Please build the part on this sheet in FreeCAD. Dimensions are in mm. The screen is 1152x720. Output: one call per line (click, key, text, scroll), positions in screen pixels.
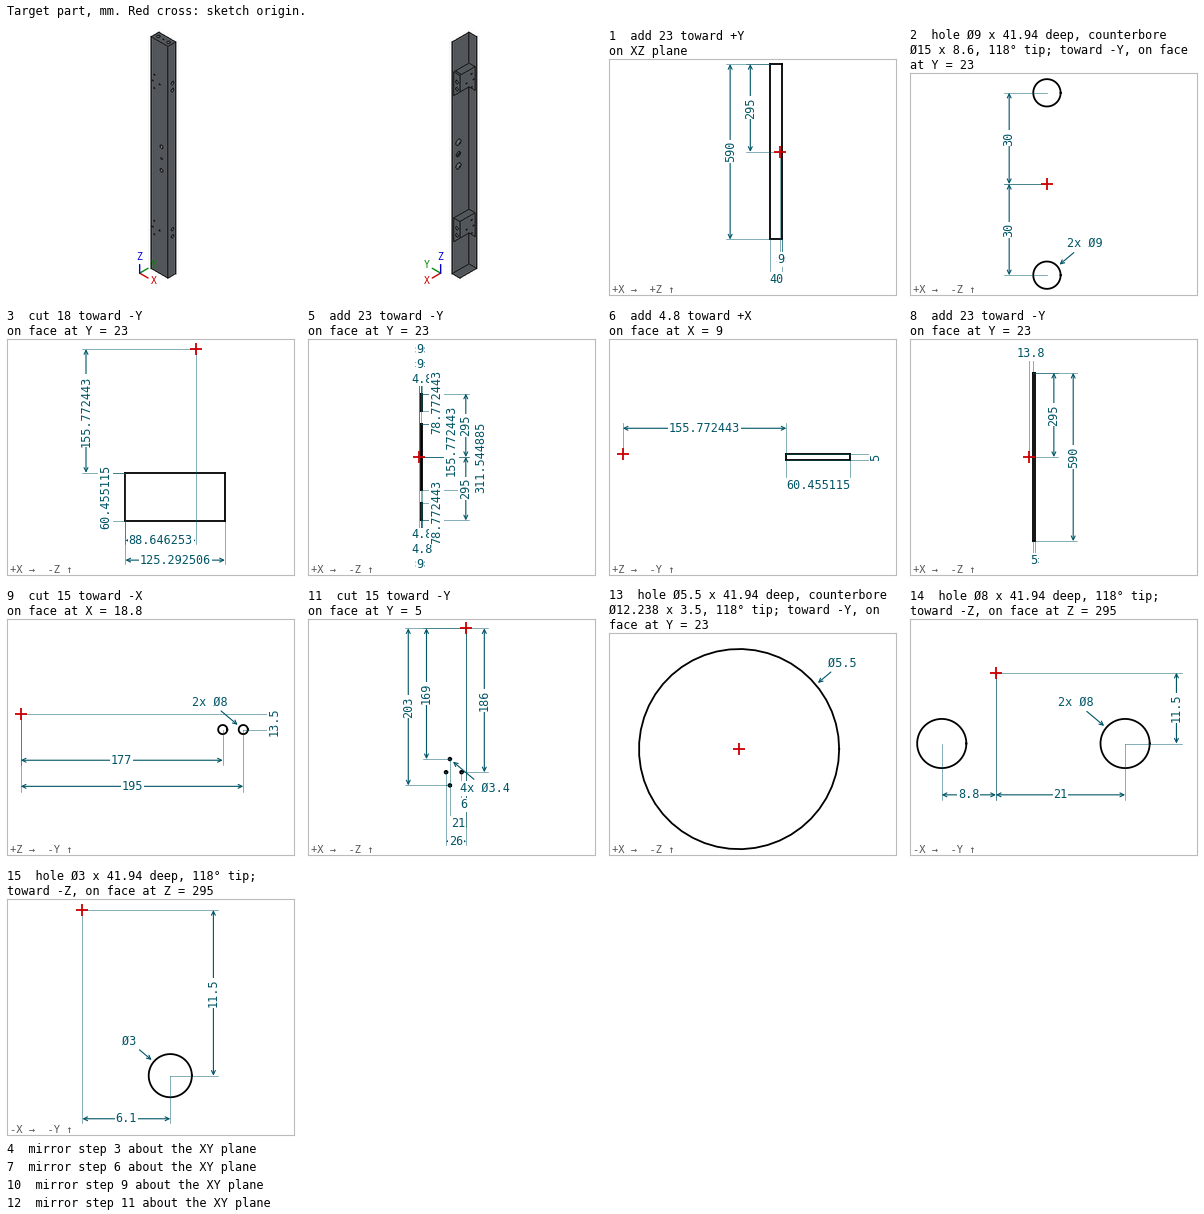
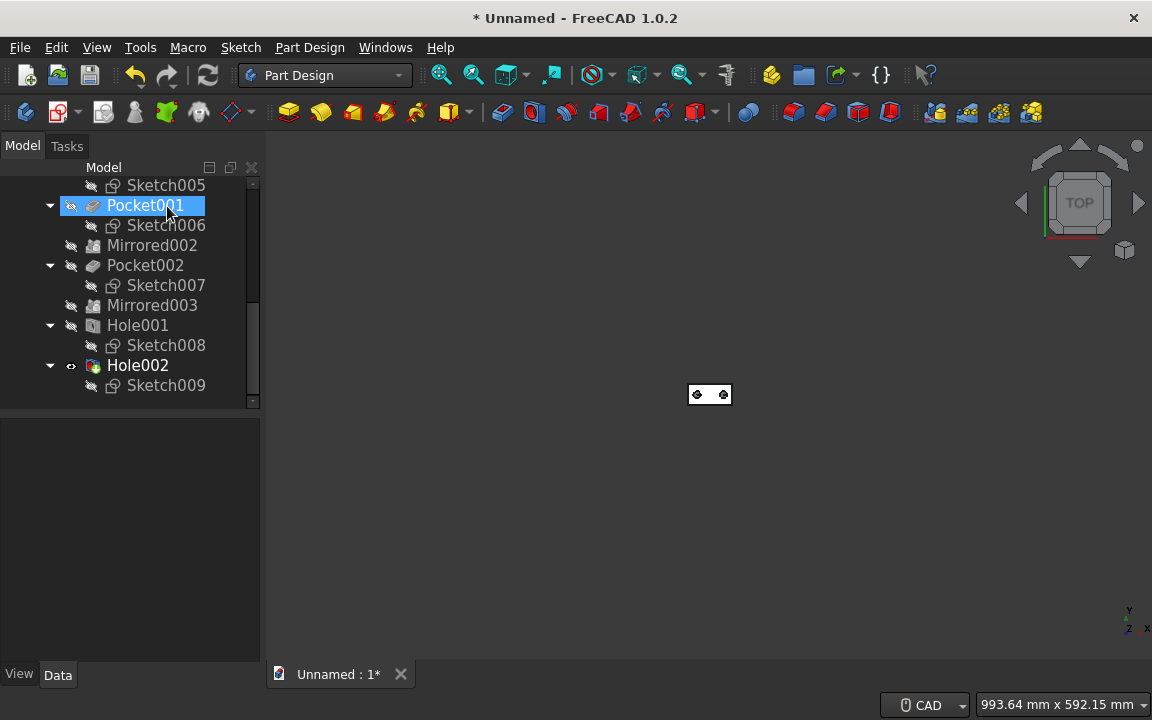
click(442, 76)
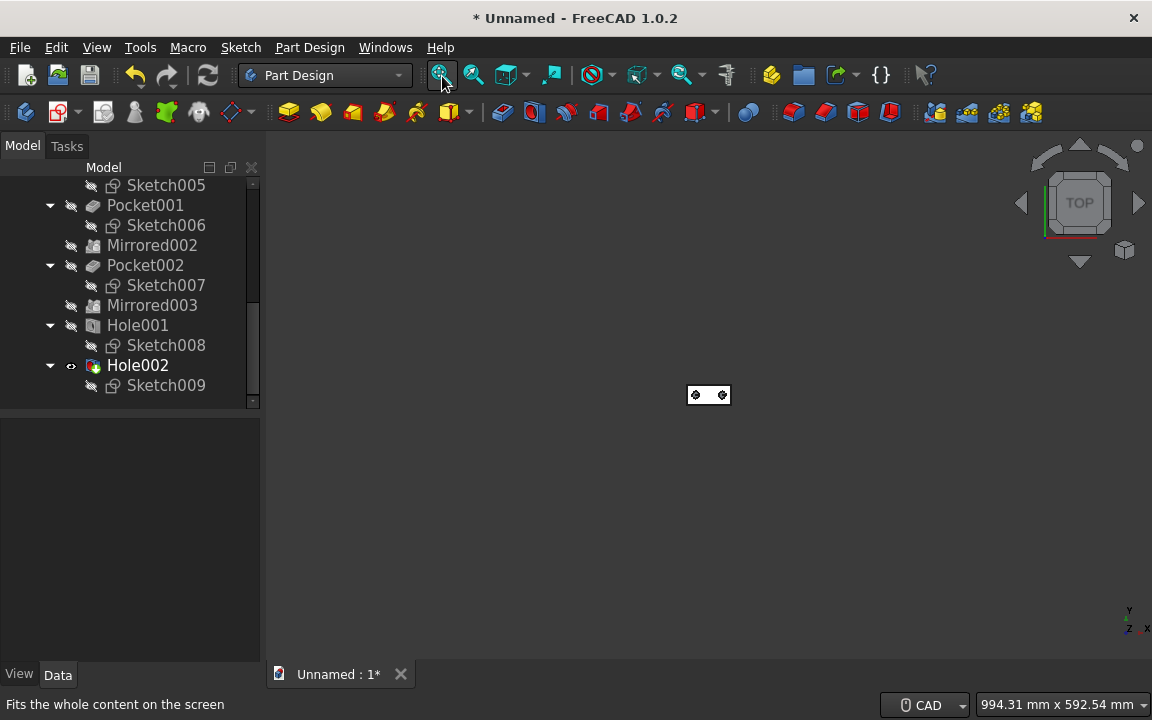
click(709, 394)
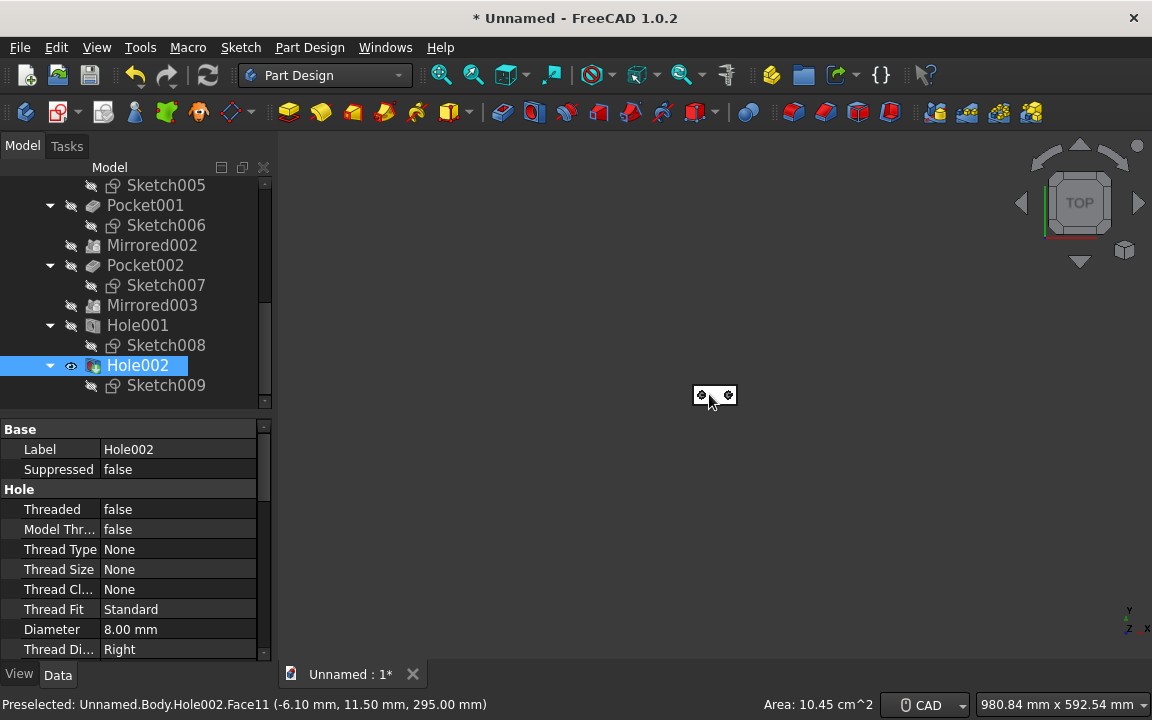
click(58, 112)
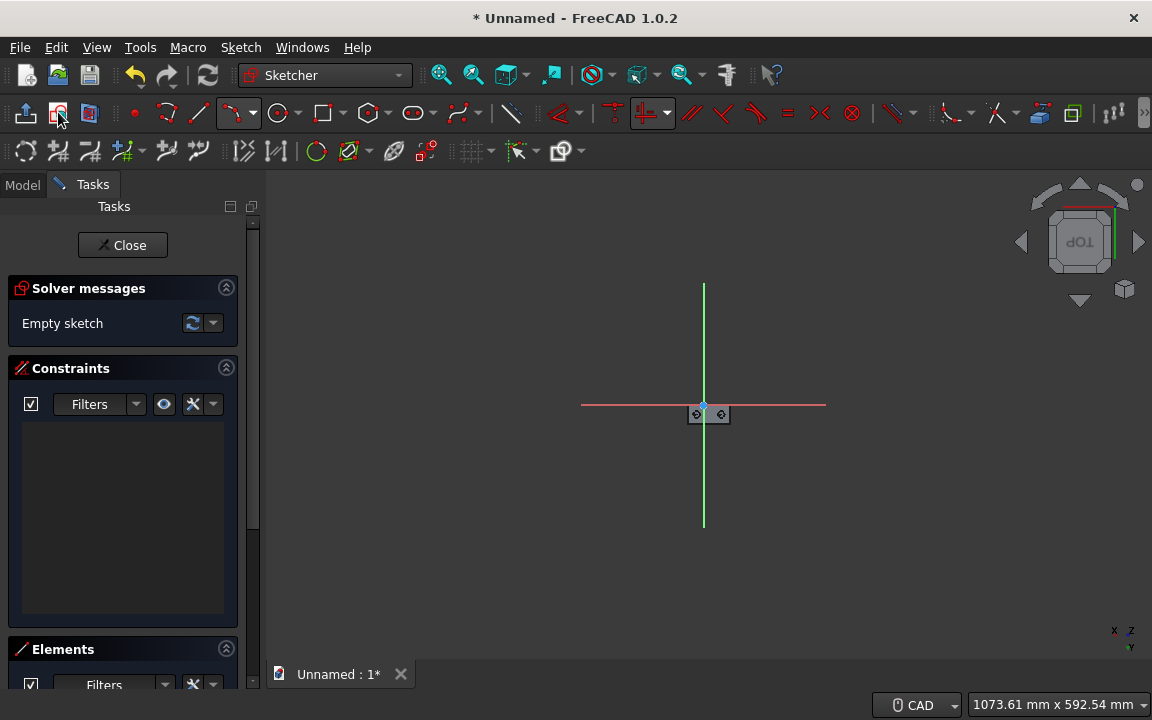
scroll(713, 414, up, 15)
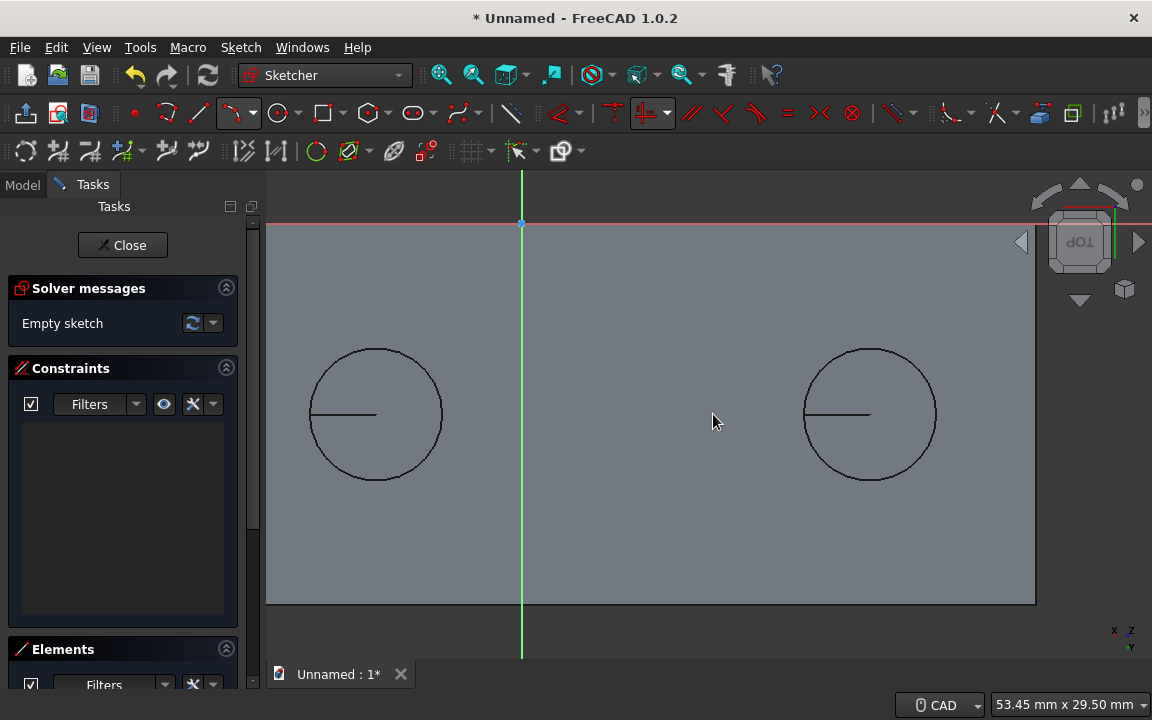
scroll(620, 414, up, 9)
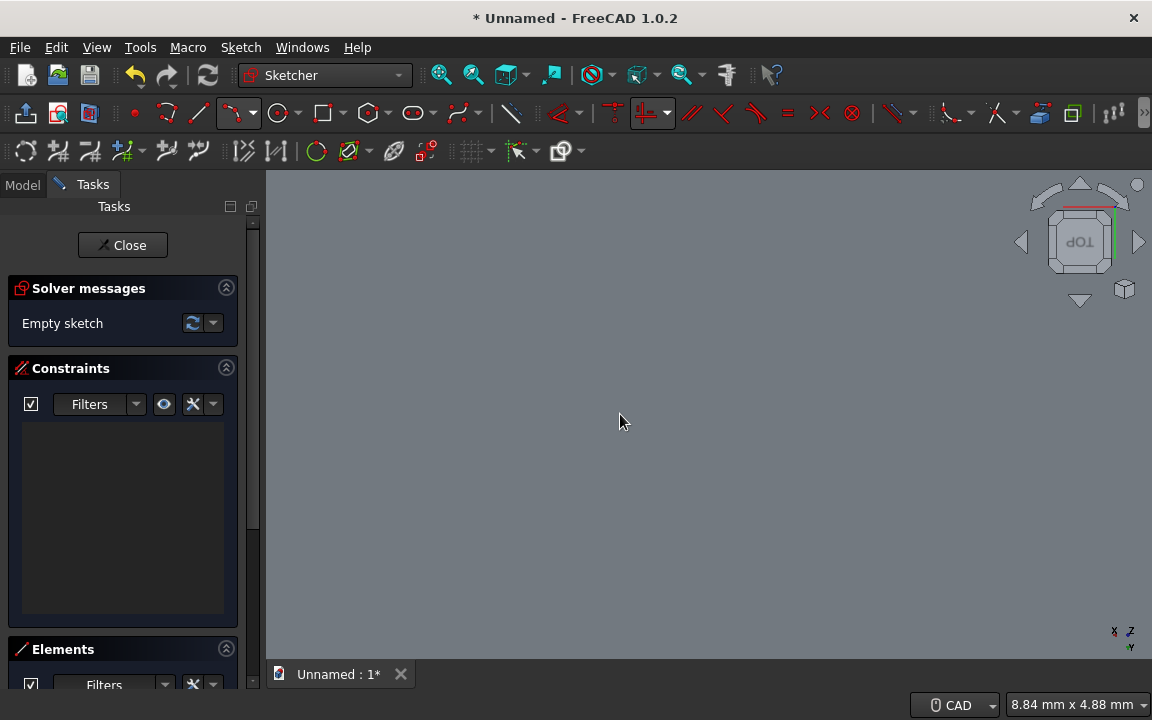
click(278, 114)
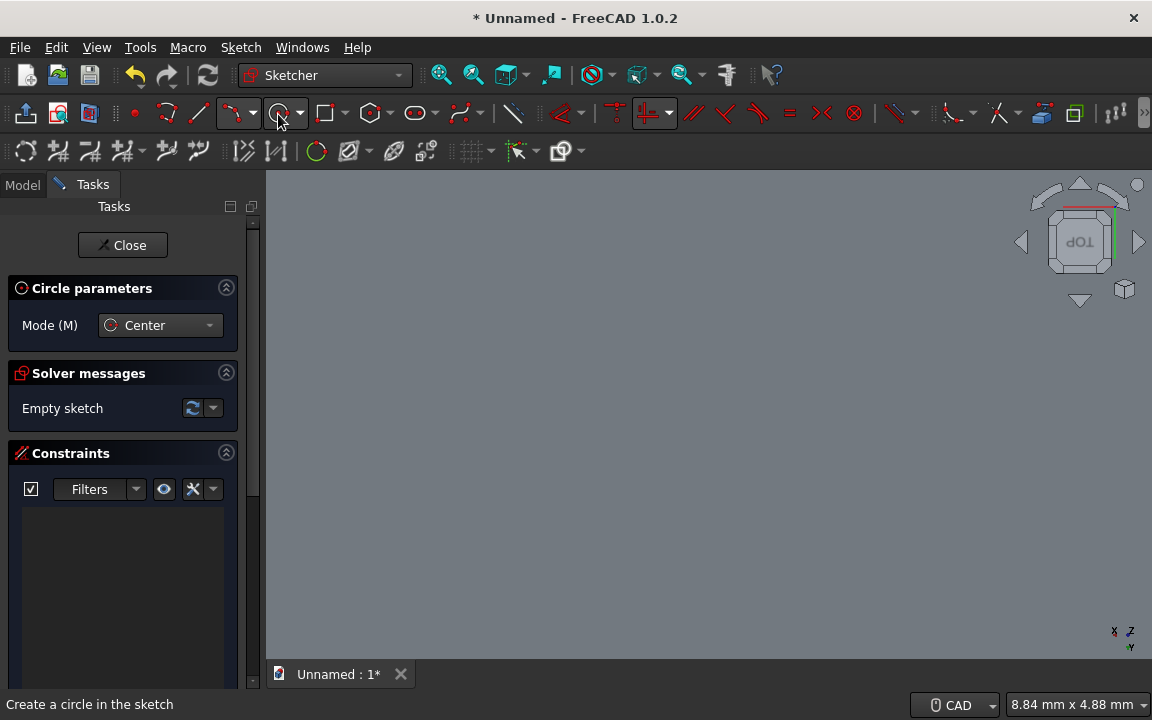
click(636, 414)
click(743, 308)
key(Escape)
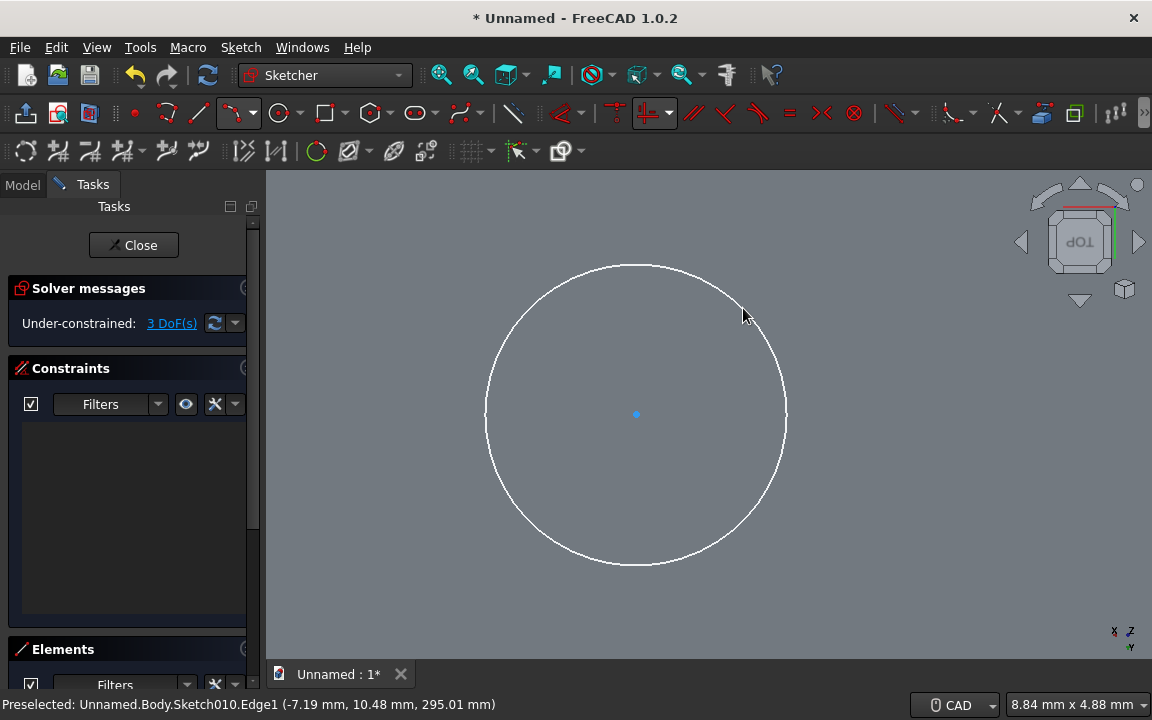
click(560, 114)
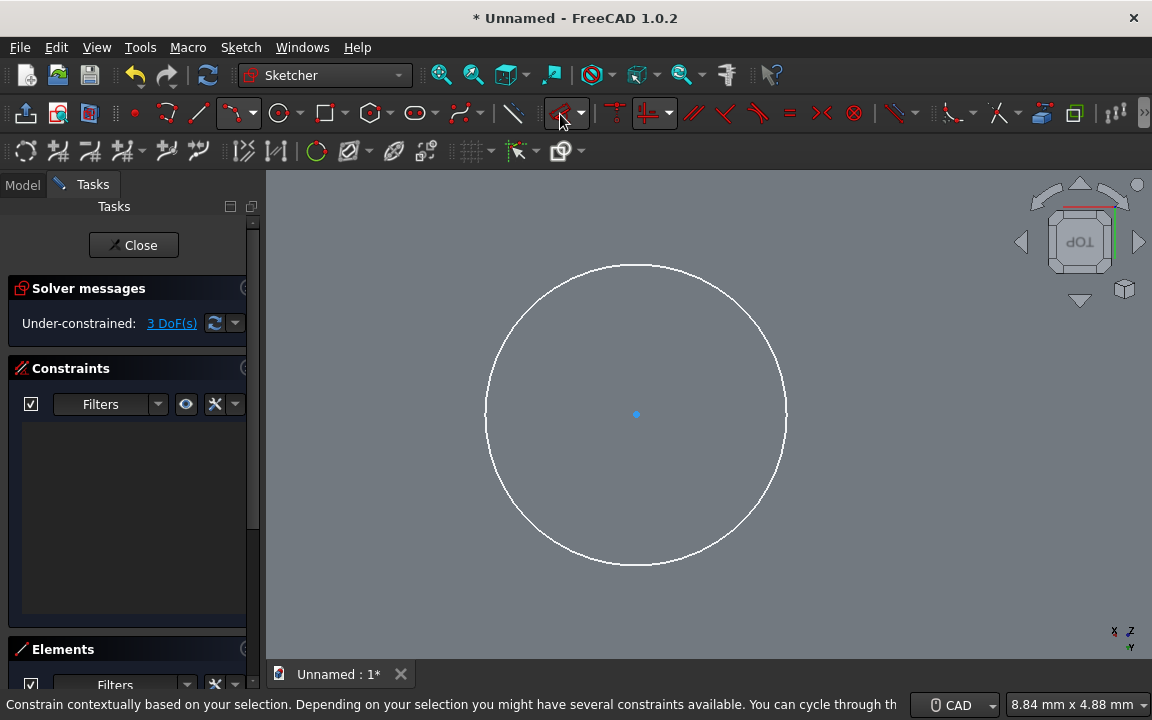
click(742, 308)
click(765, 285)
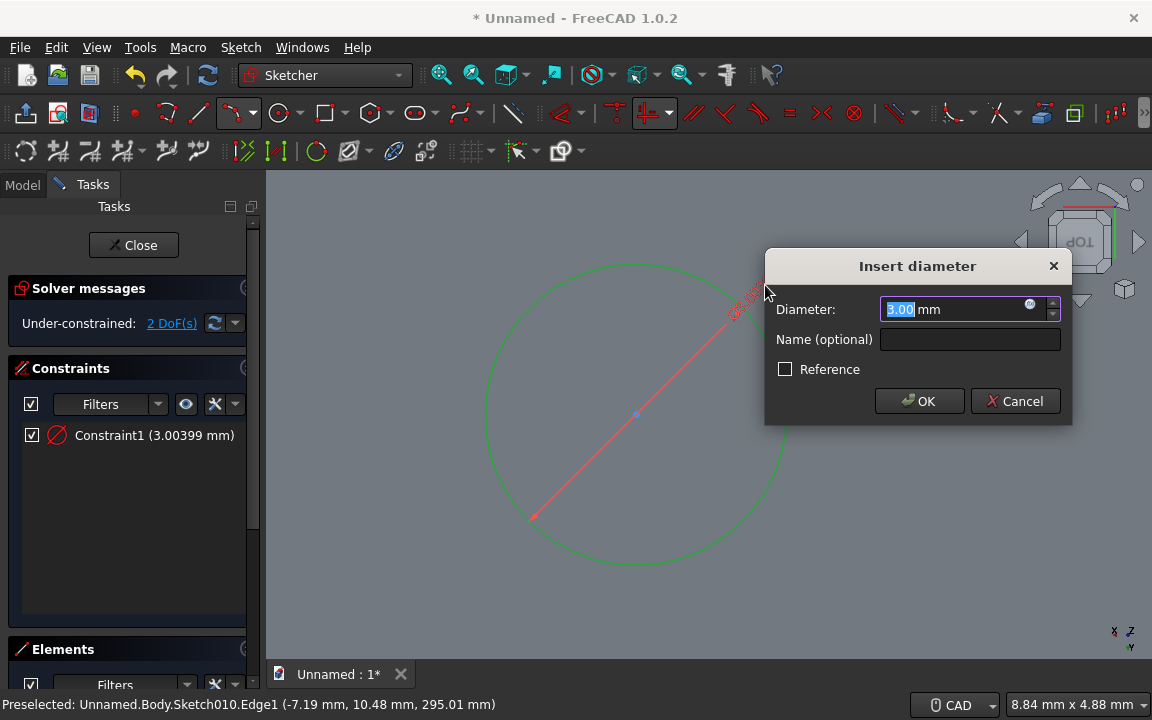
text(3)
key(Return)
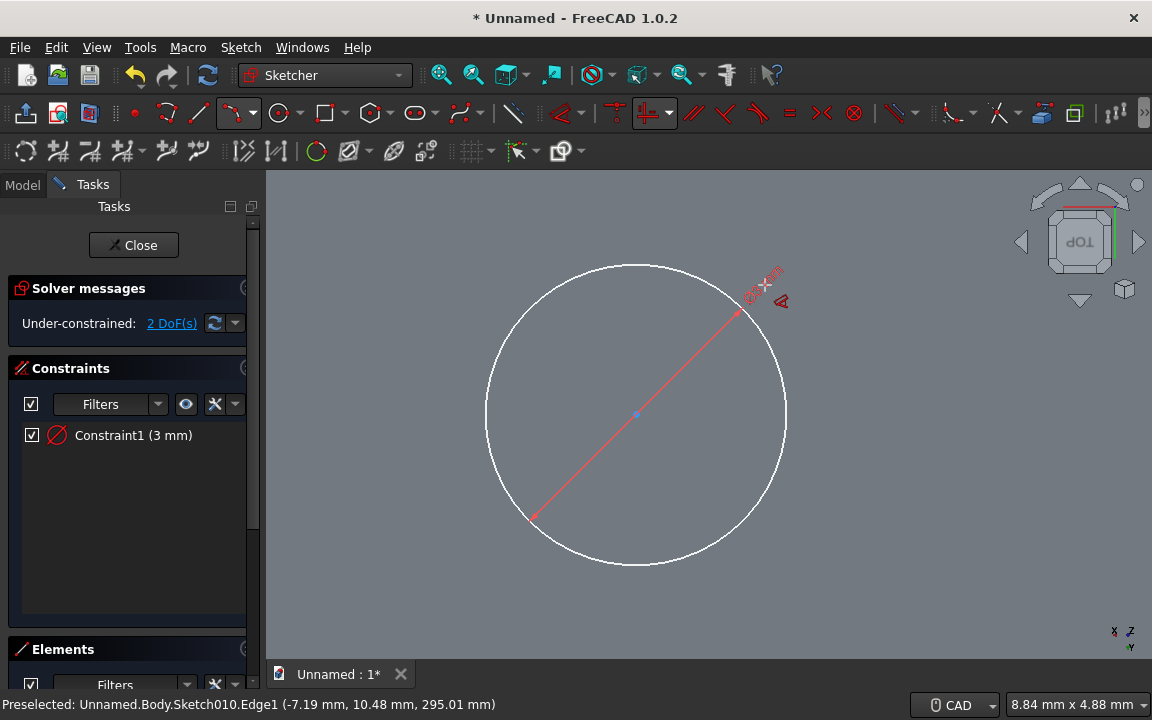
click(636, 415)
click(465, 449)